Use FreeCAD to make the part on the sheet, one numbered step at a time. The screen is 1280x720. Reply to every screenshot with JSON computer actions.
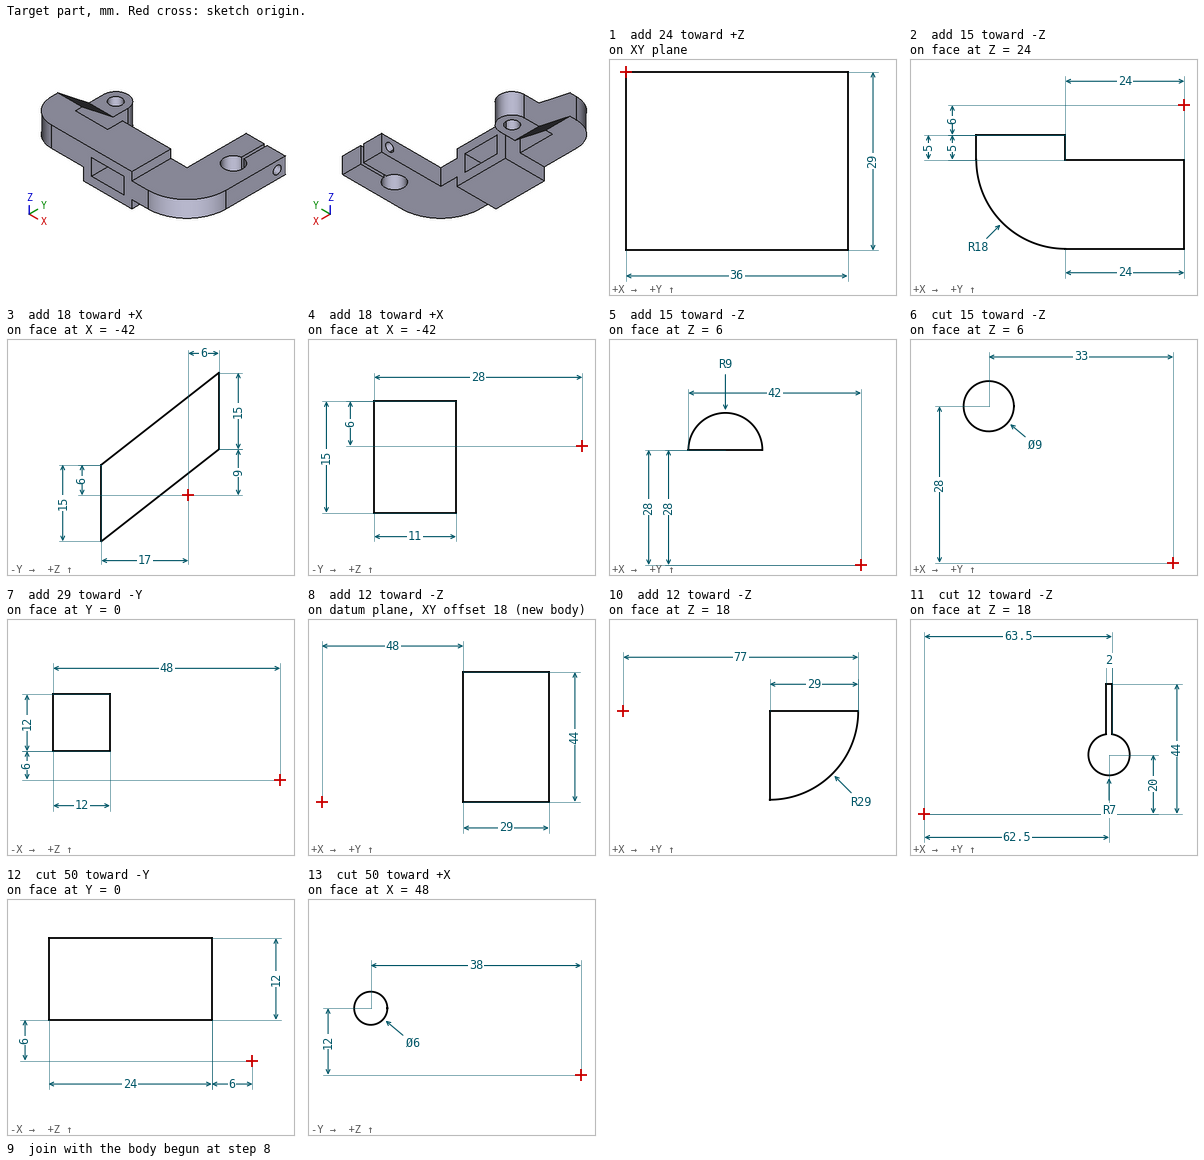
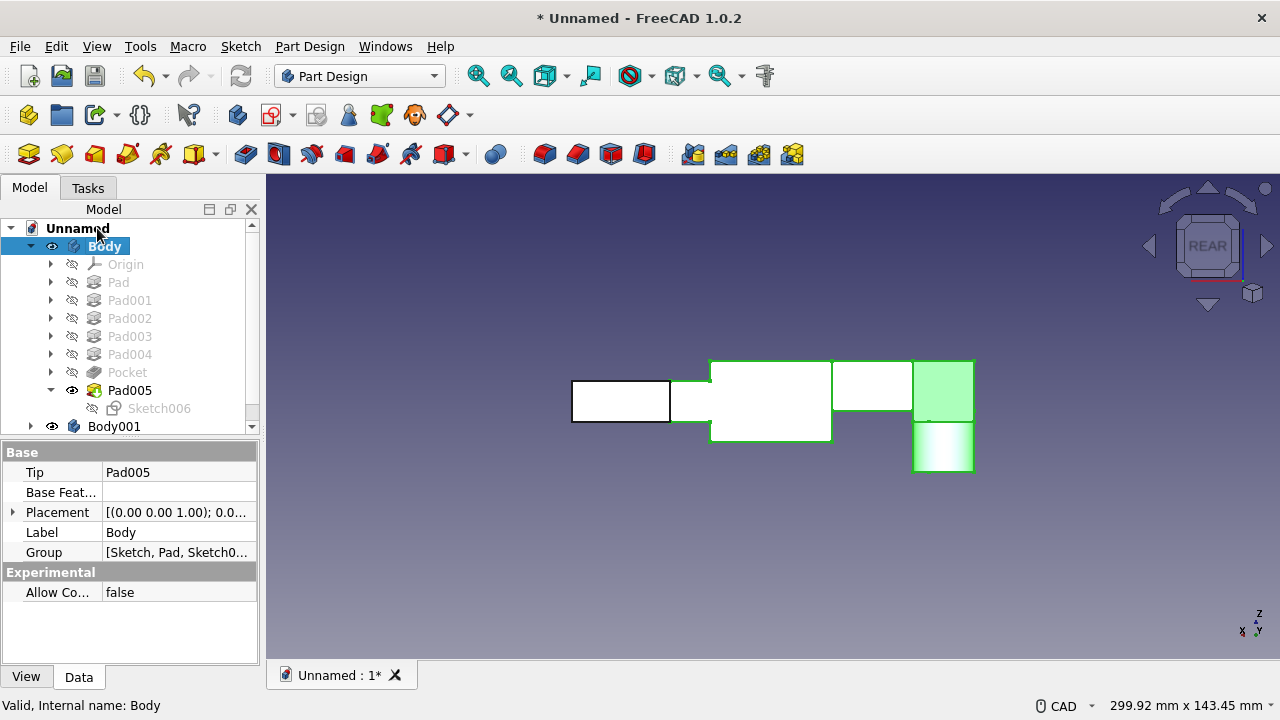
{"action": "left_click", "coordinate": [97, 246]}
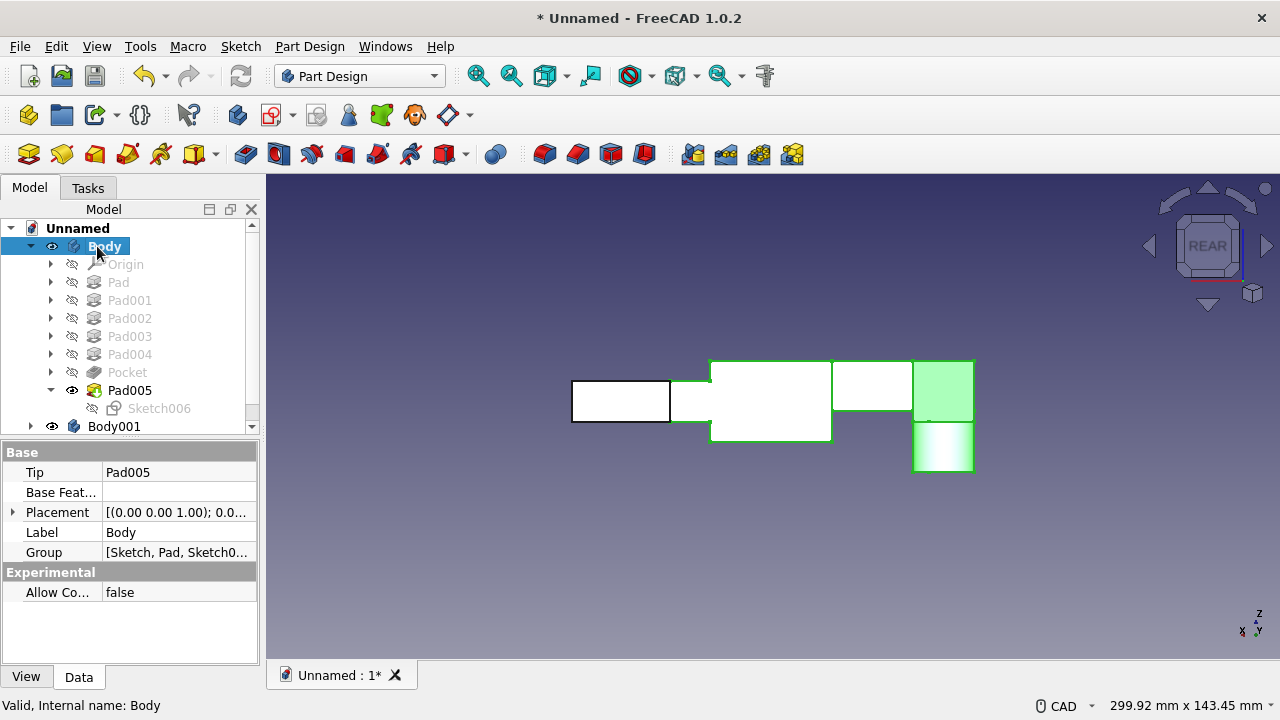
{"action": "left_click", "coordinate": [148, 592]}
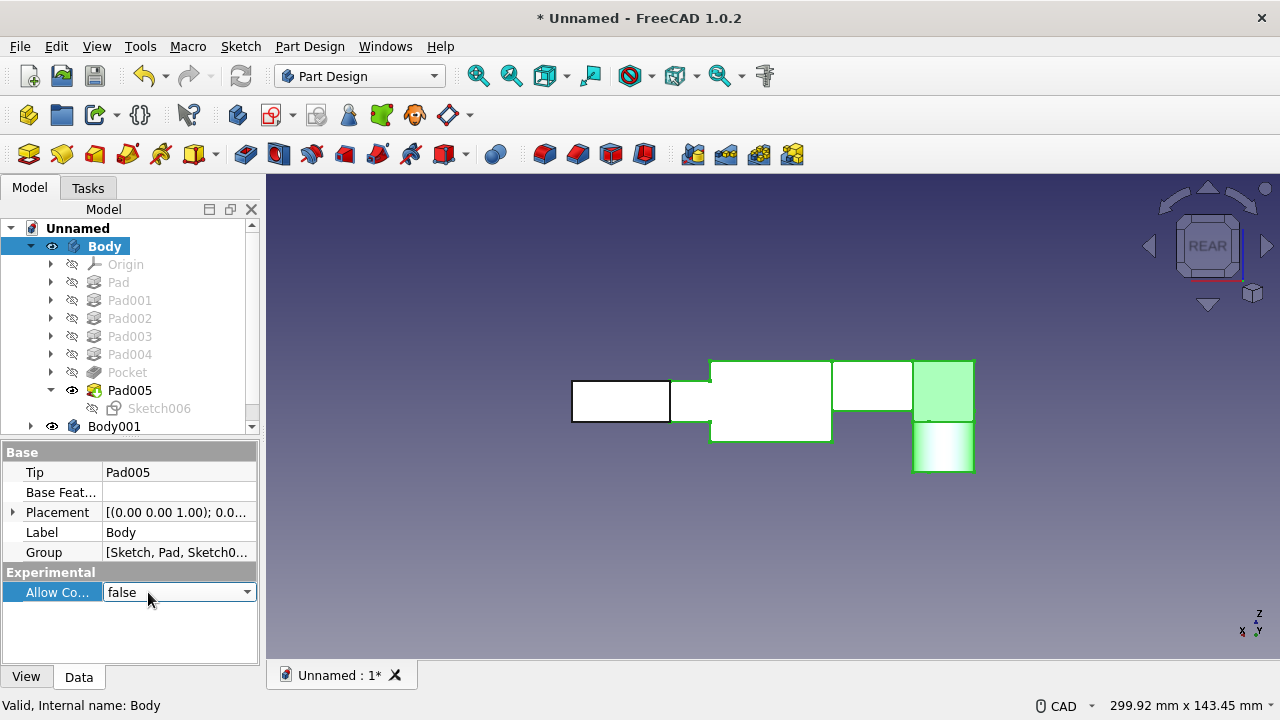
{"action": "left_click", "coordinate": [148, 592]}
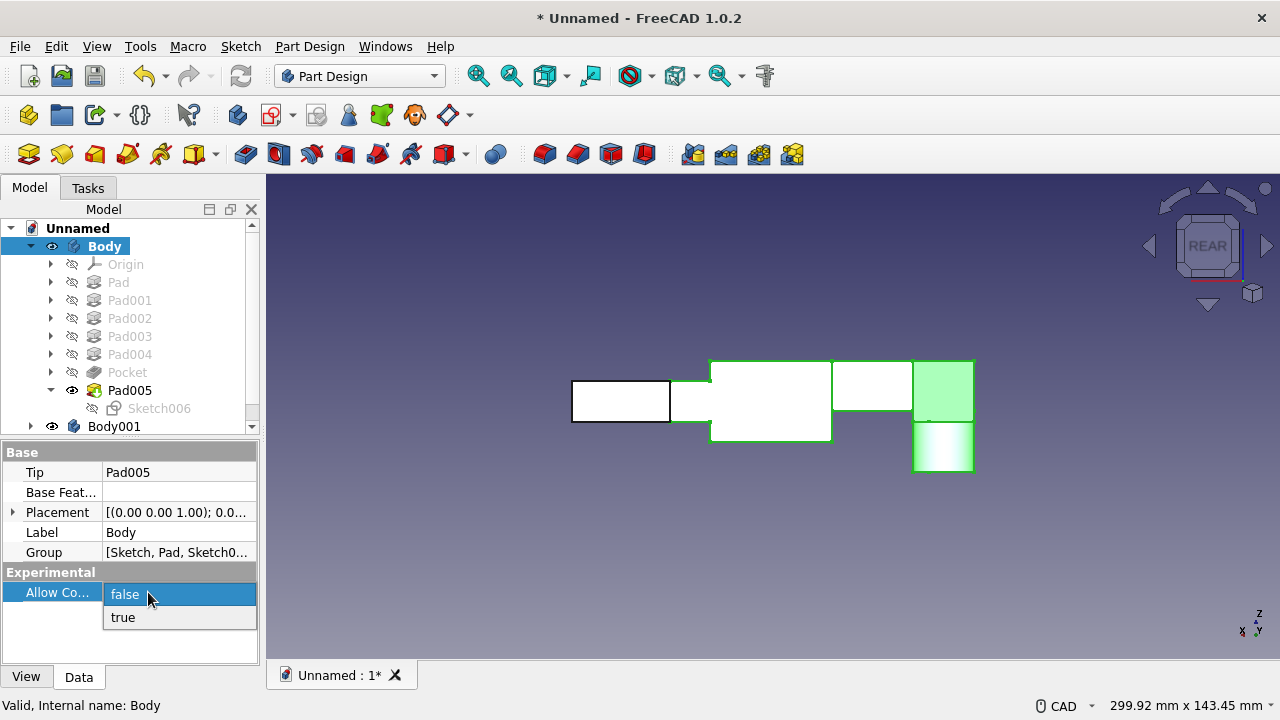
{"action": "left_click", "coordinate": [178, 618]}
{"action": "key", "text": "Return"}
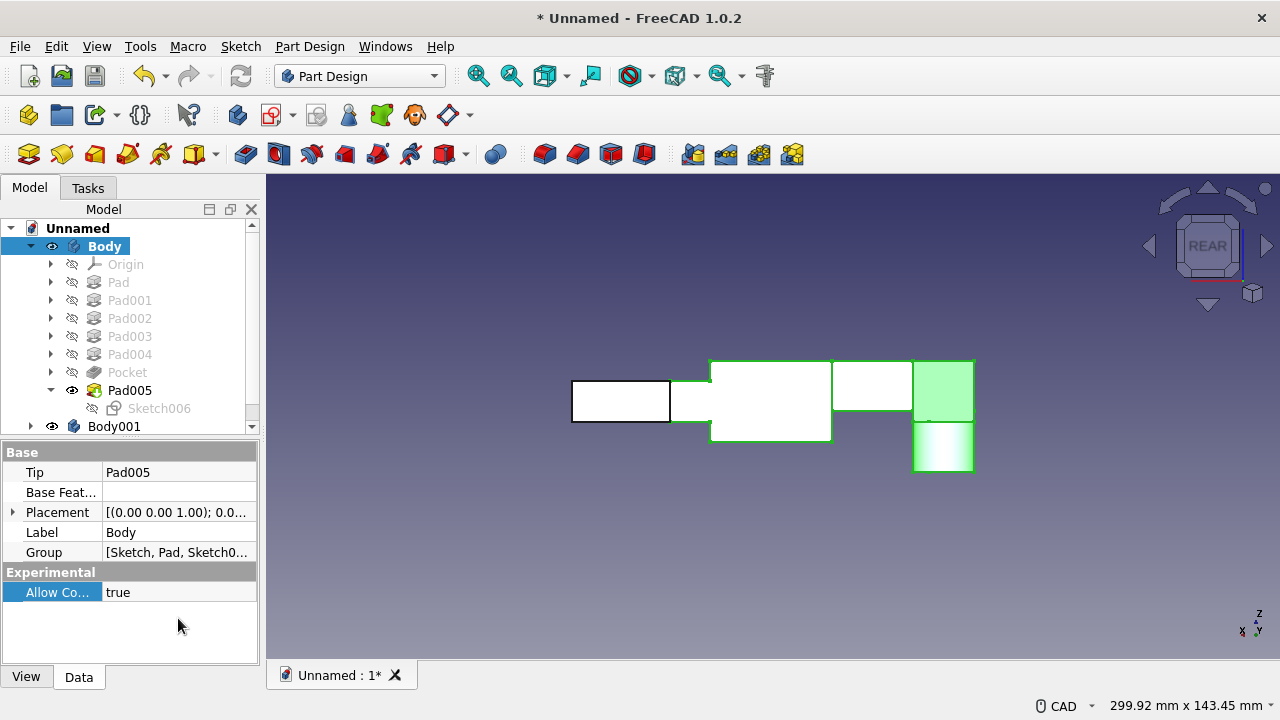
{"action": "left_click", "coordinate": [97, 426]}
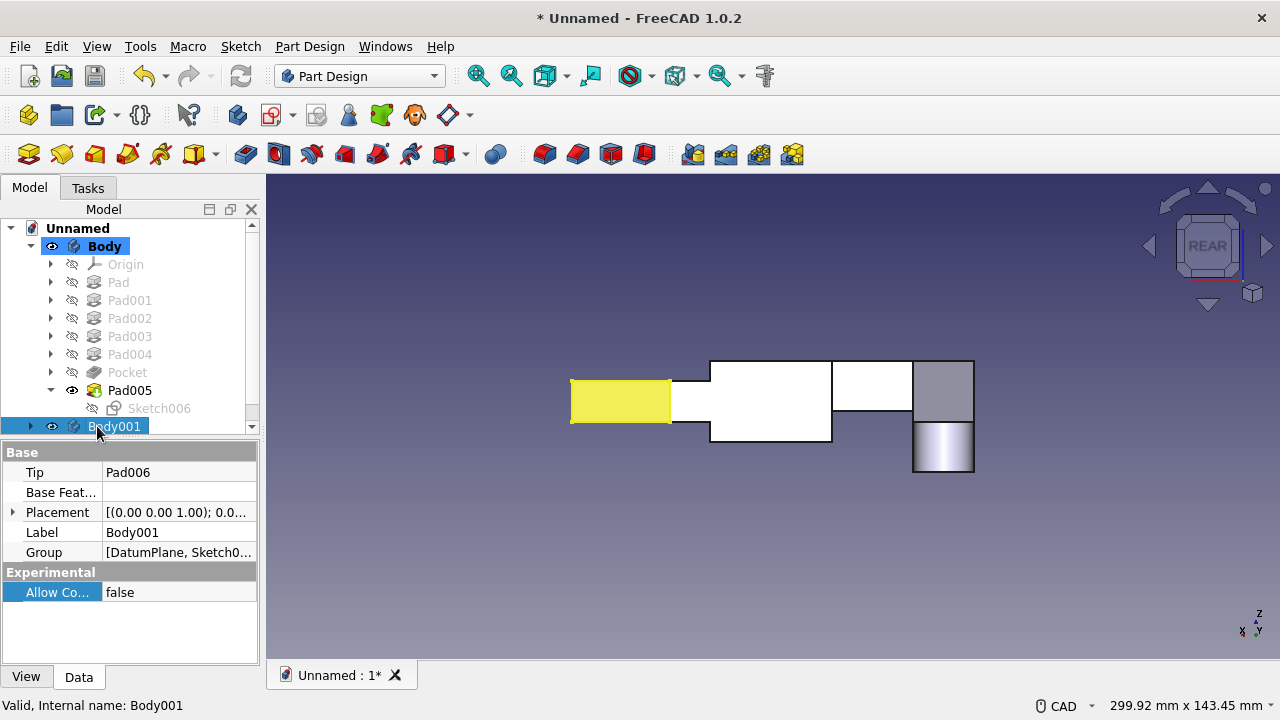
{"action": "left_click", "coordinate": [496, 154]}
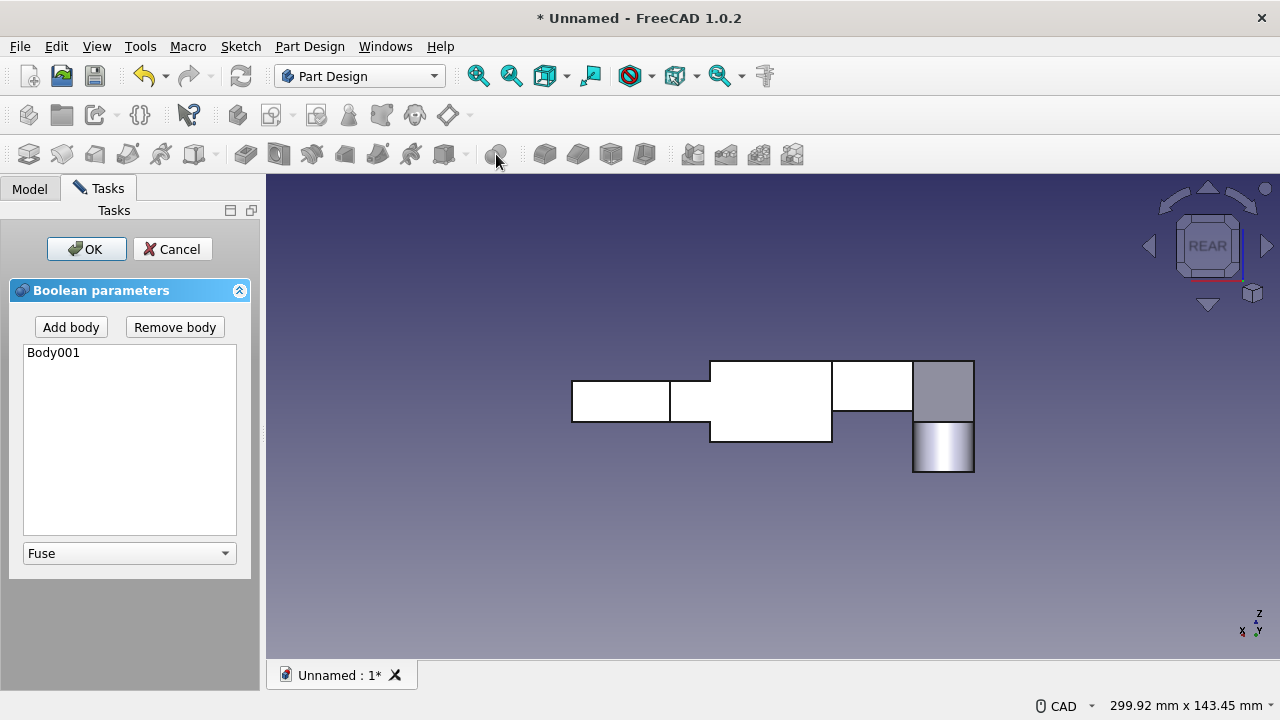
{"action": "left_click", "coordinate": [87, 249]}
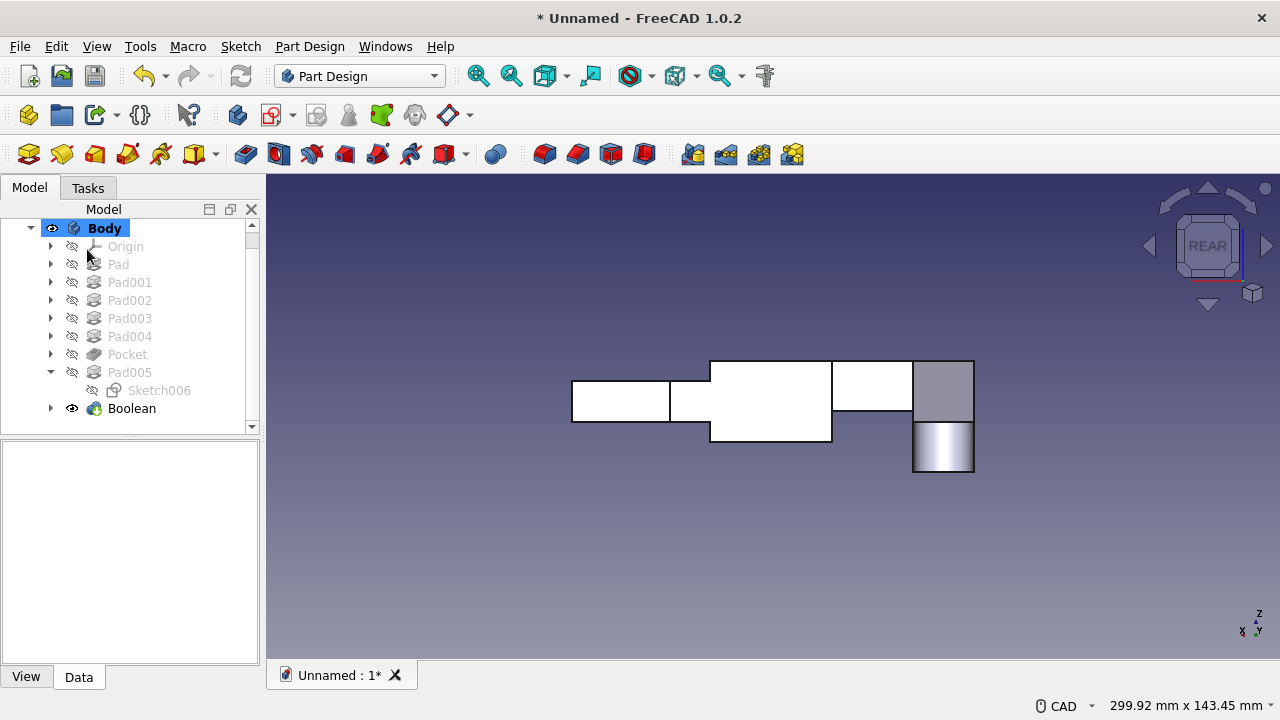
{"action": "left_click", "coordinate": [479, 76]}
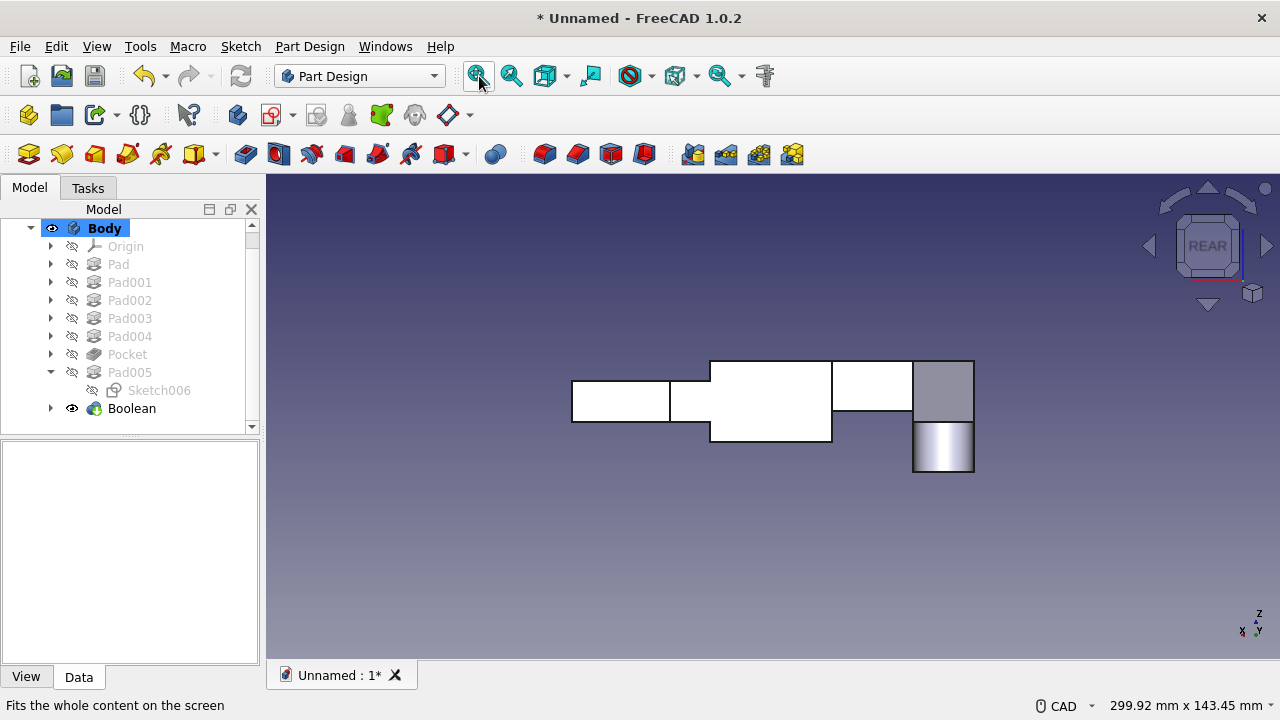
{"action": "key", "text": "0"}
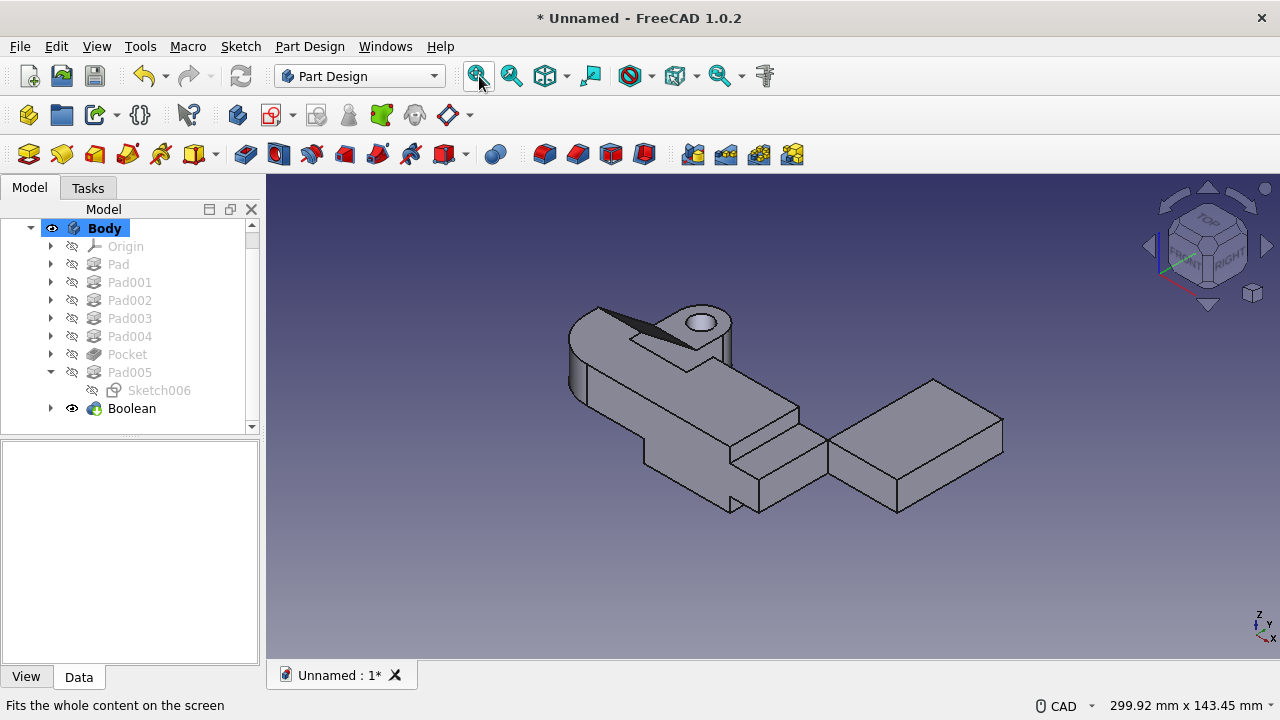
{"action": "left_click", "coordinate": [930, 420]}